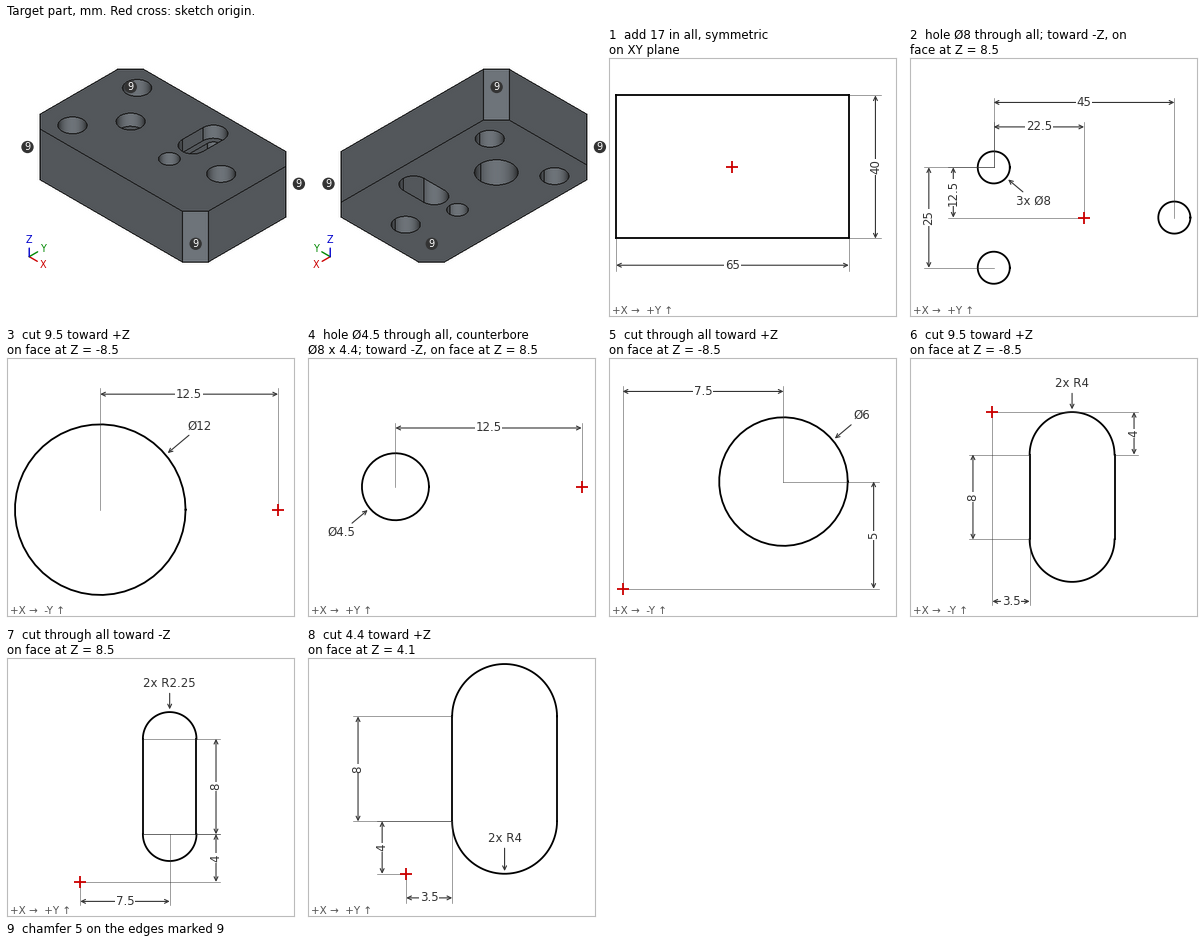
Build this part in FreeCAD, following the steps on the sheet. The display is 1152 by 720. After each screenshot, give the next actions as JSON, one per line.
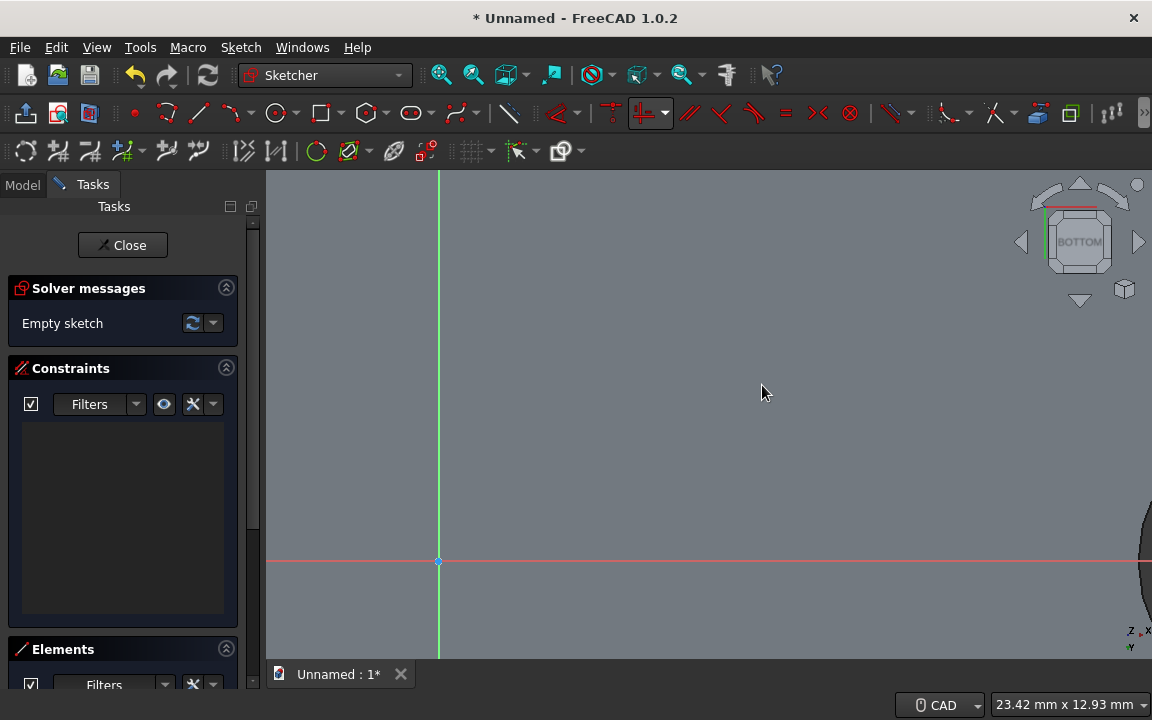
{"action": "left_click", "coordinate": [276, 114]}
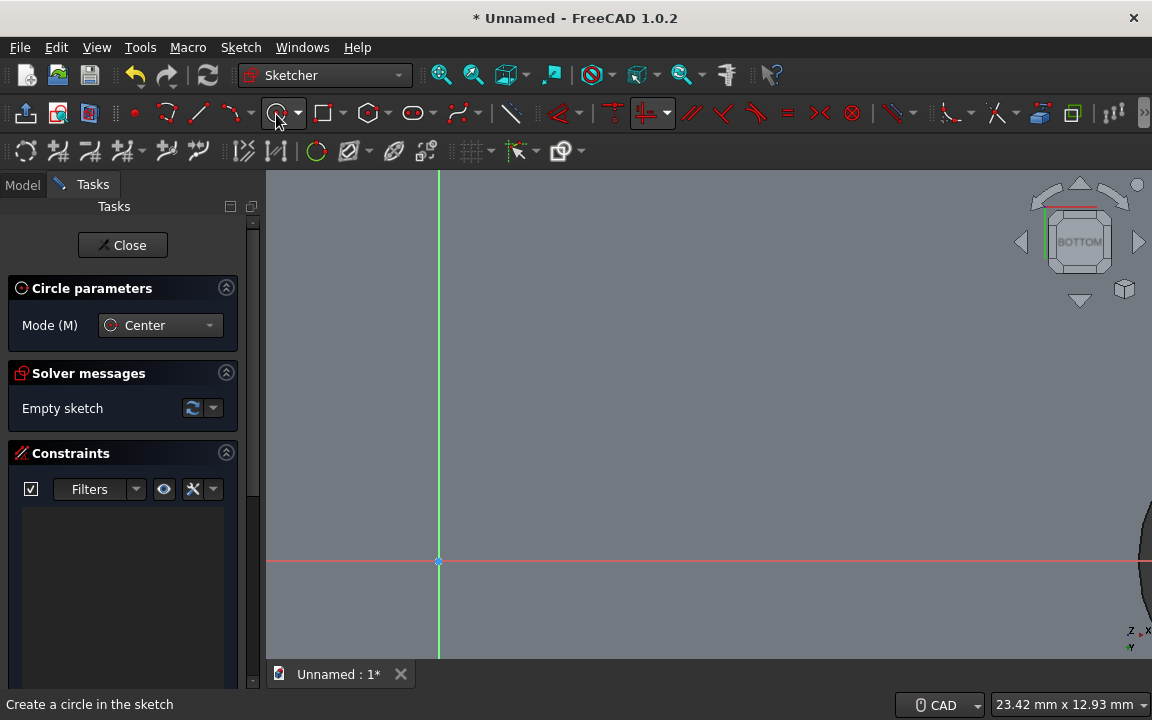
{"action": "left_click", "coordinate": [722, 372]}
{"action": "left_click", "coordinate": [803, 292]}
{"action": "key", "text": "Escape"}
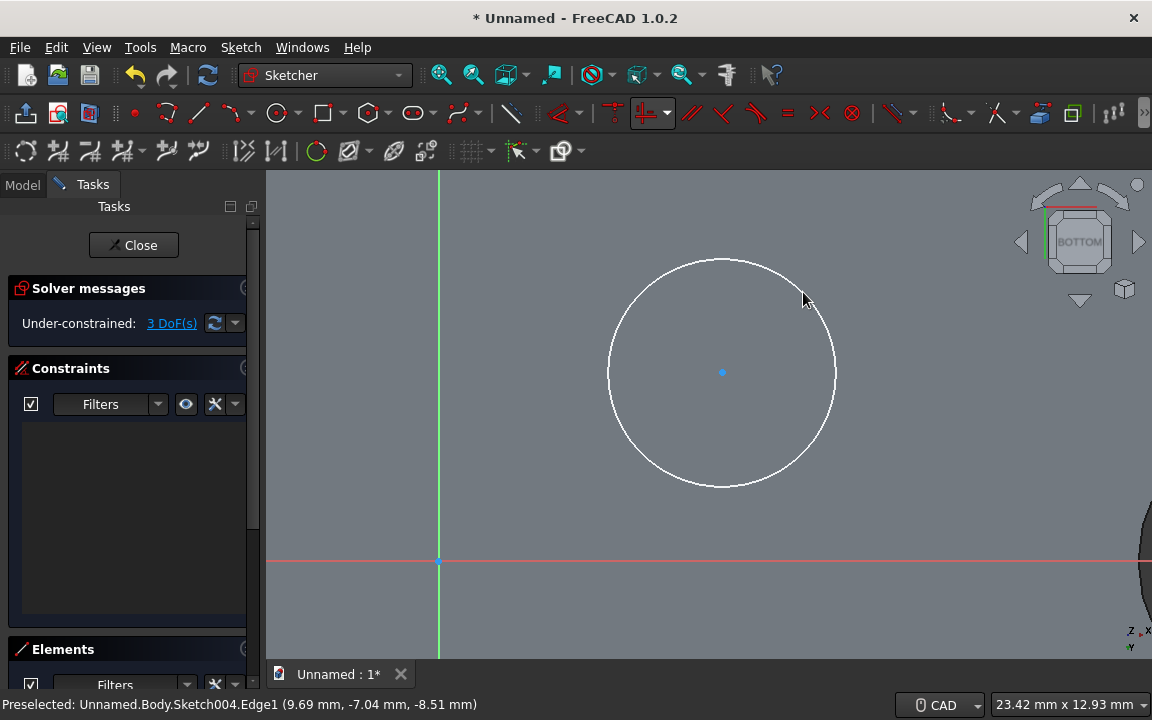
{"action": "left_click", "coordinate": [558, 114]}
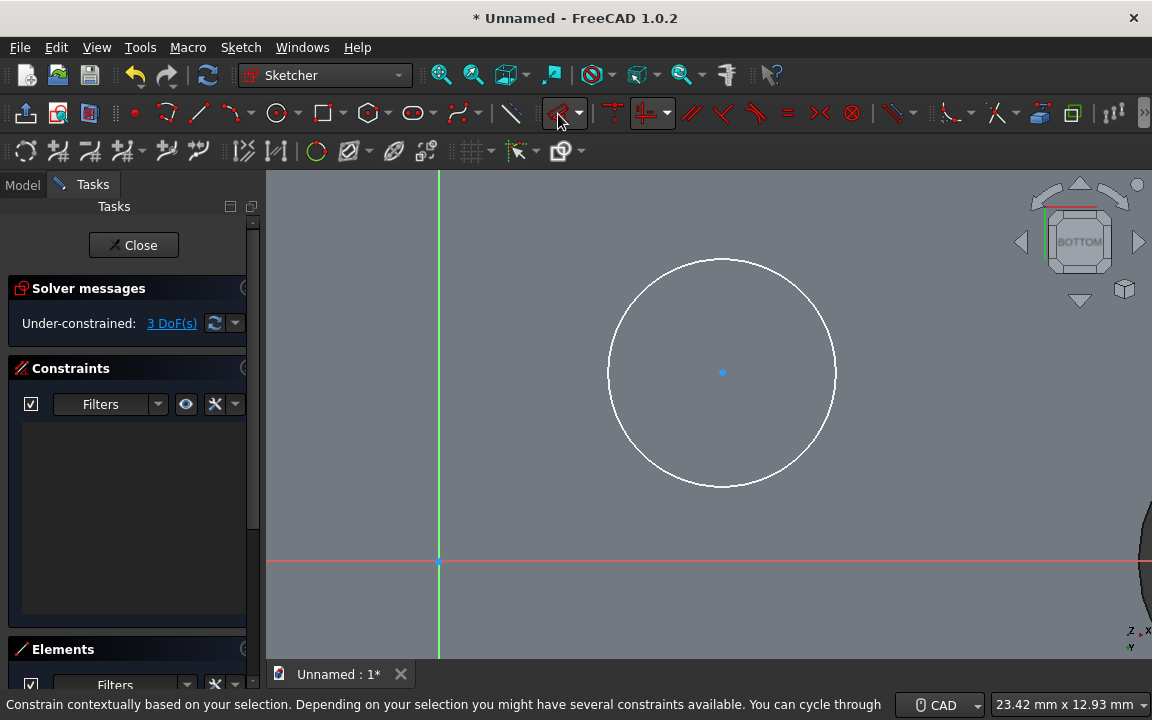
{"action": "left_click", "coordinate": [802, 292]}
{"action": "left_click", "coordinate": [824, 269]}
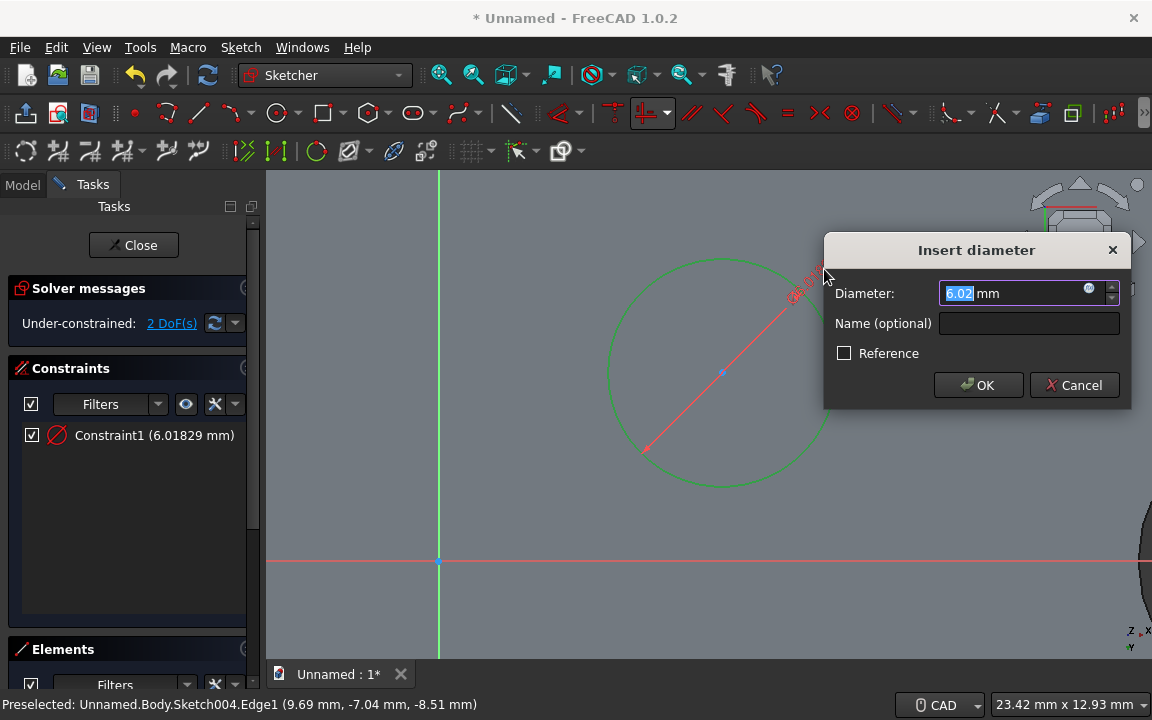
{"action": "type", "text": "6"}
{"action": "key", "text": "Return"}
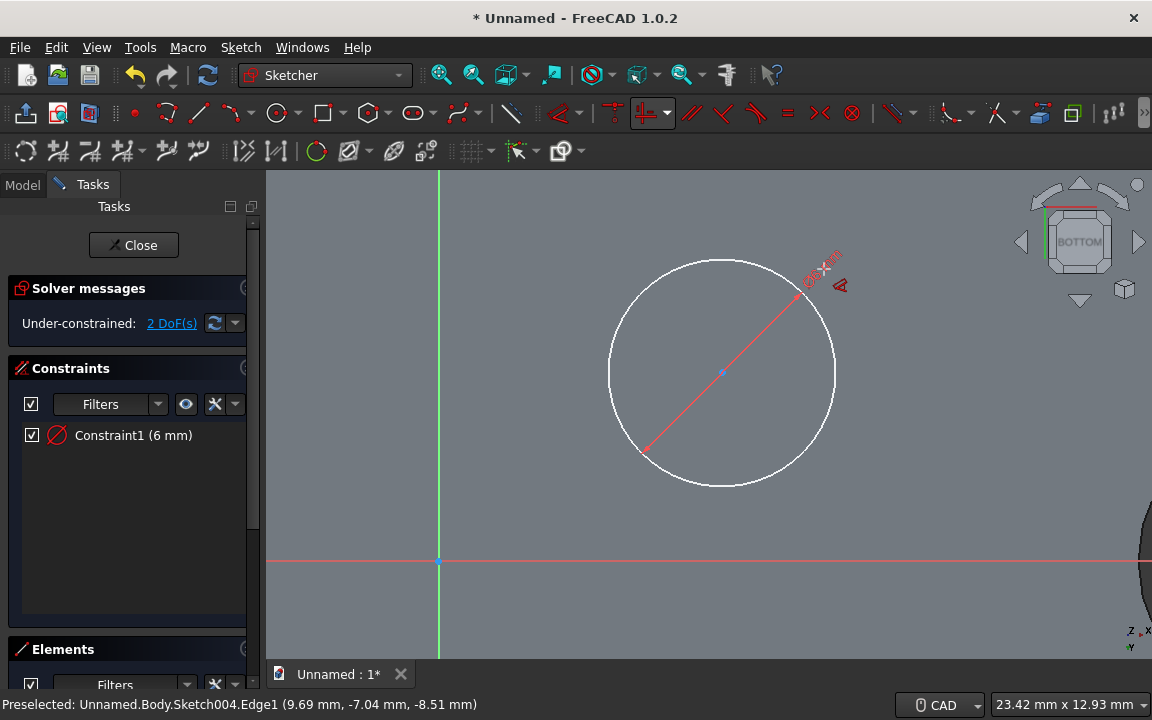
{"action": "left_click", "coordinate": [722, 373]}
{"action": "left_click", "coordinate": [405, 467]}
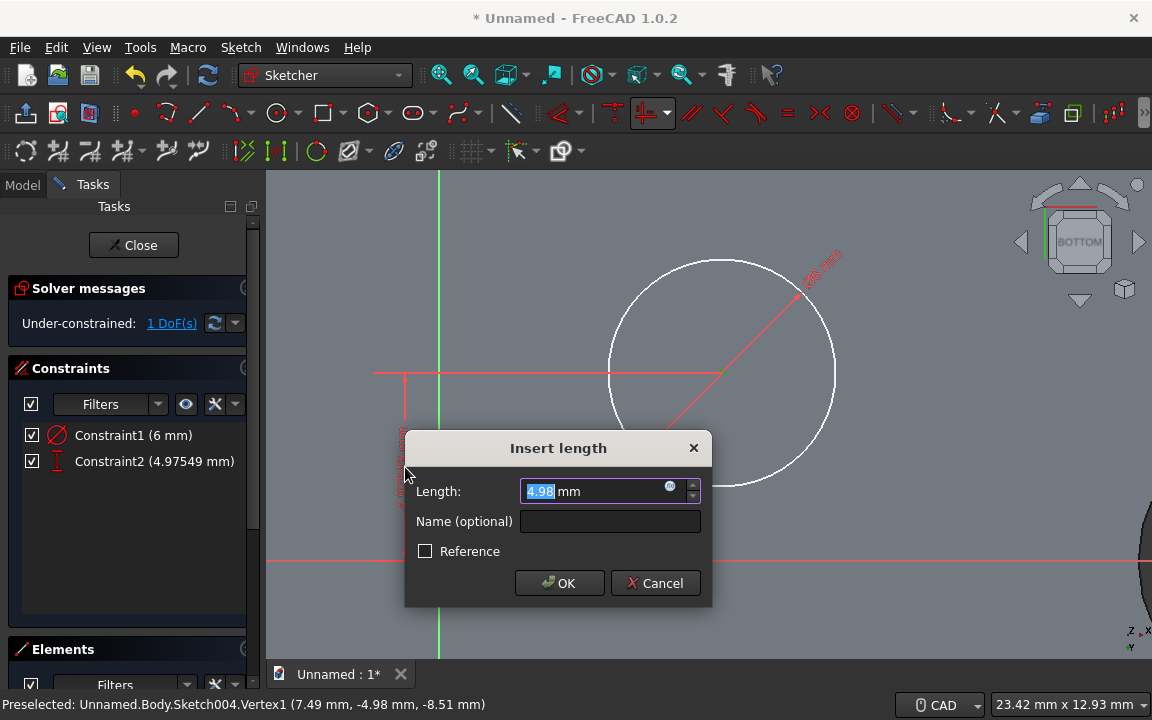
{"action": "type", "text": "5"}
{"action": "key", "text": "Return"}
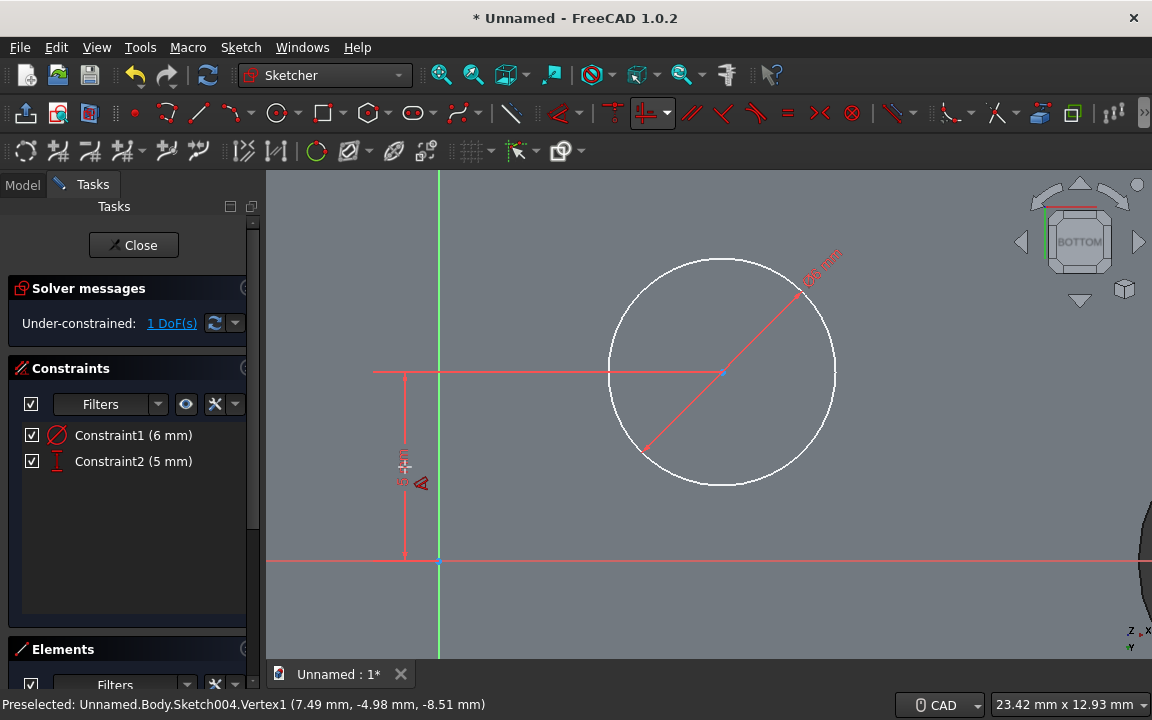
{"action": "left_click", "coordinate": [722, 372]}
{"action": "left_click", "coordinate": [580, 595]}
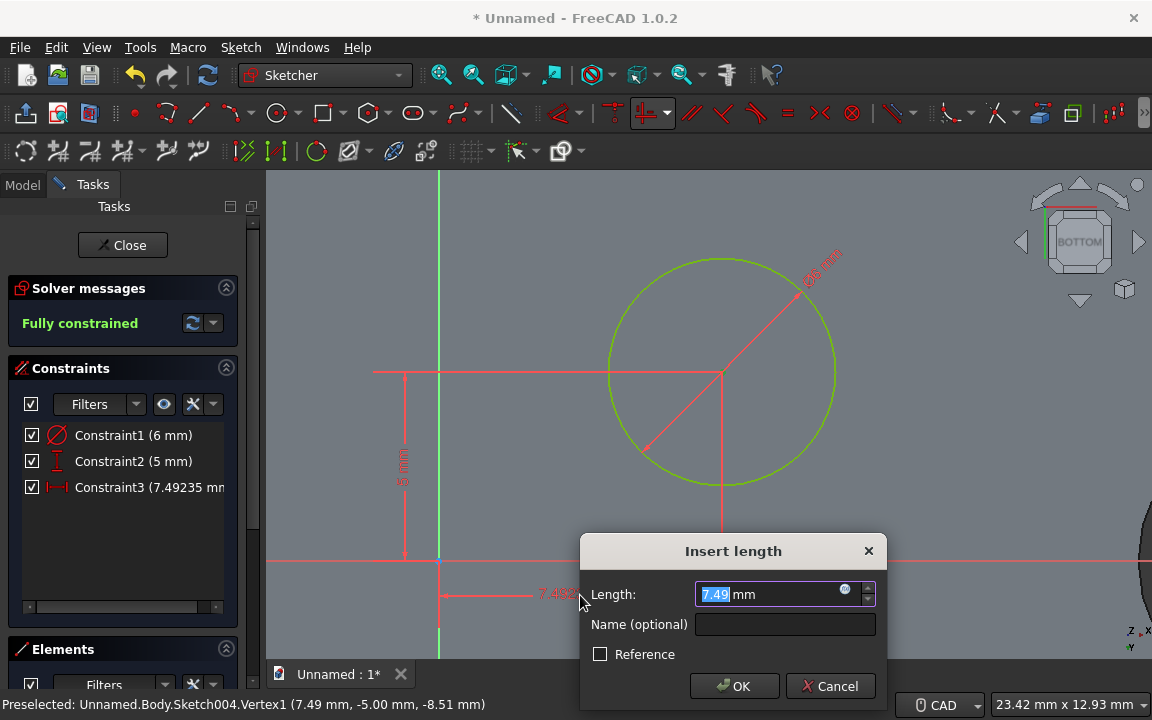
{"action": "type", "text": "7.5"}
{"action": "key", "text": "Return"}
{"action": "key", "text": "Escape"}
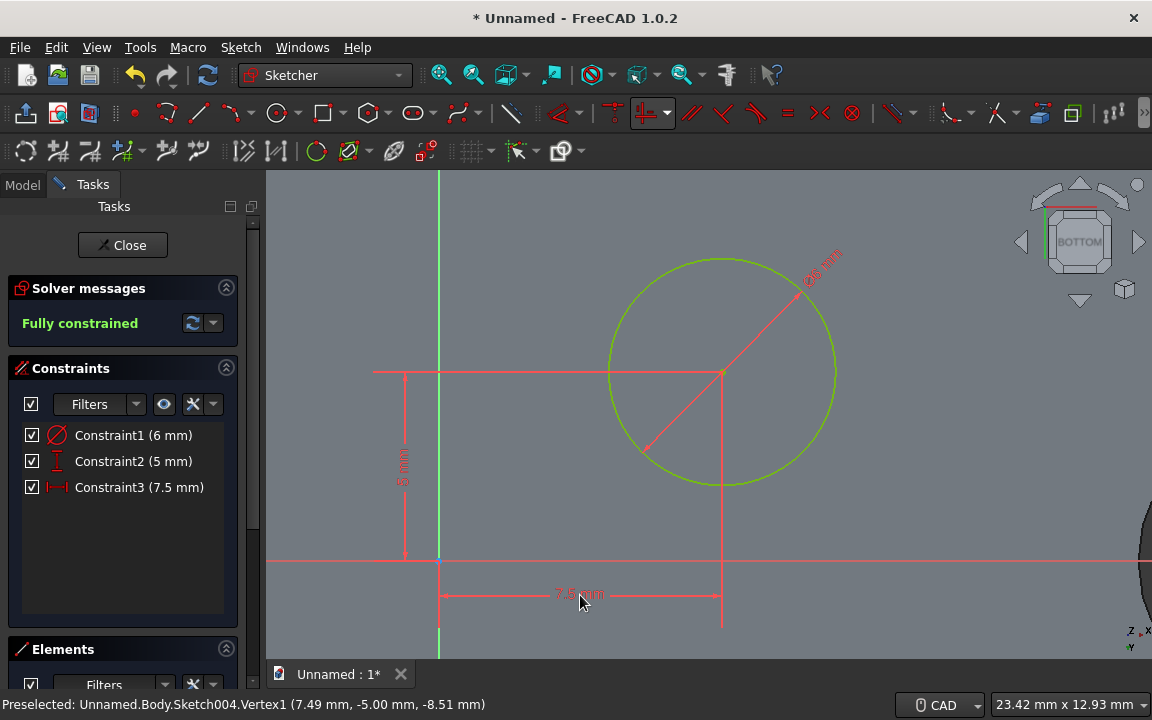
{"action": "left_click", "coordinate": [123, 245]}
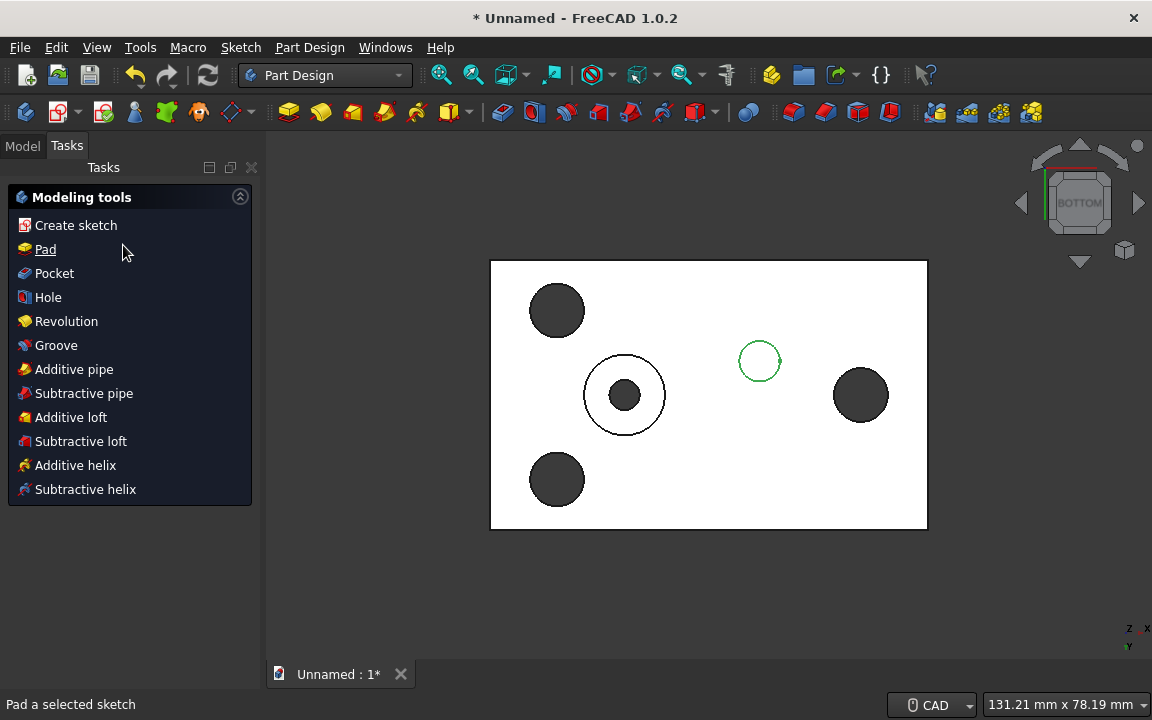
{"action": "left_click", "coordinate": [504, 112]}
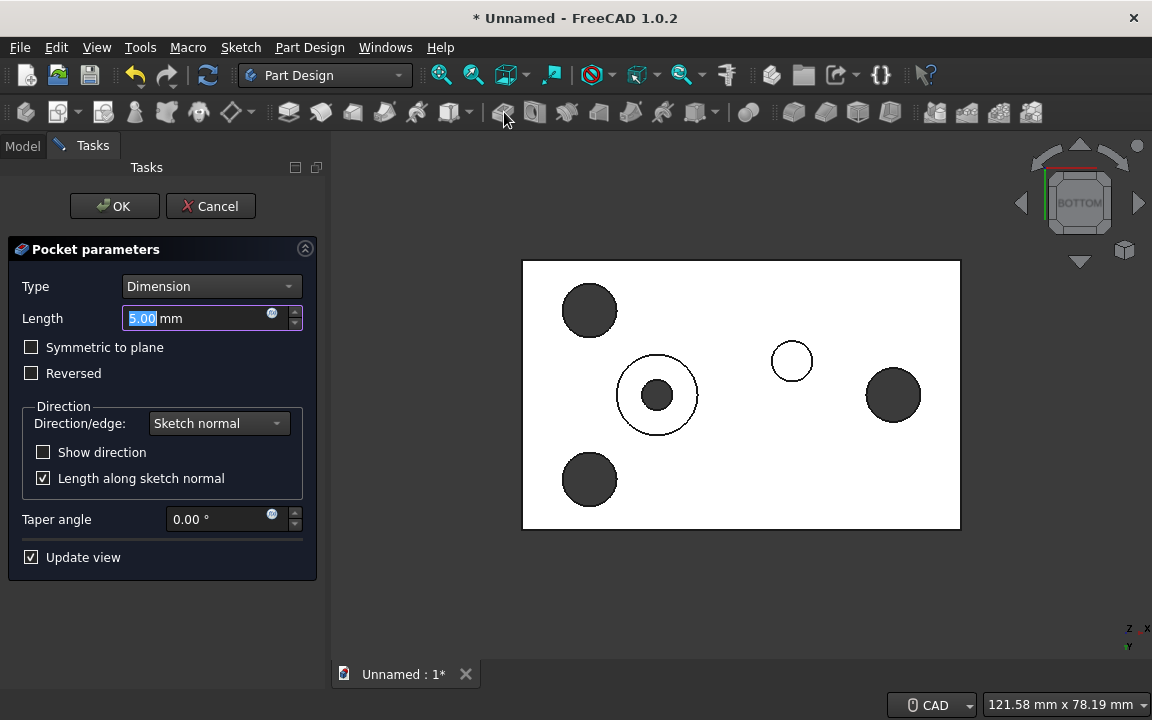
{"action": "left_click", "coordinate": [212, 286]}